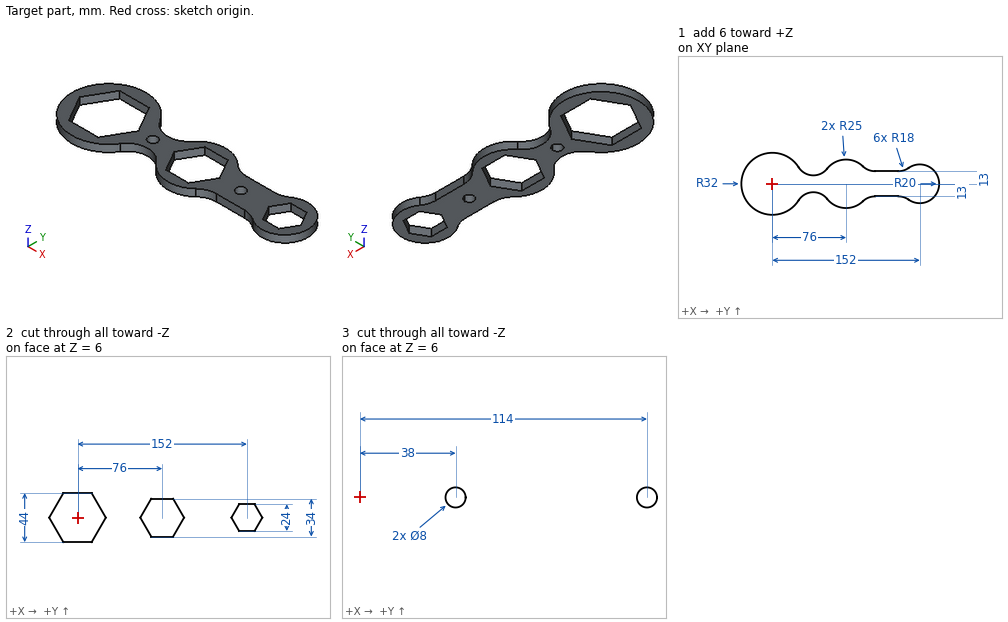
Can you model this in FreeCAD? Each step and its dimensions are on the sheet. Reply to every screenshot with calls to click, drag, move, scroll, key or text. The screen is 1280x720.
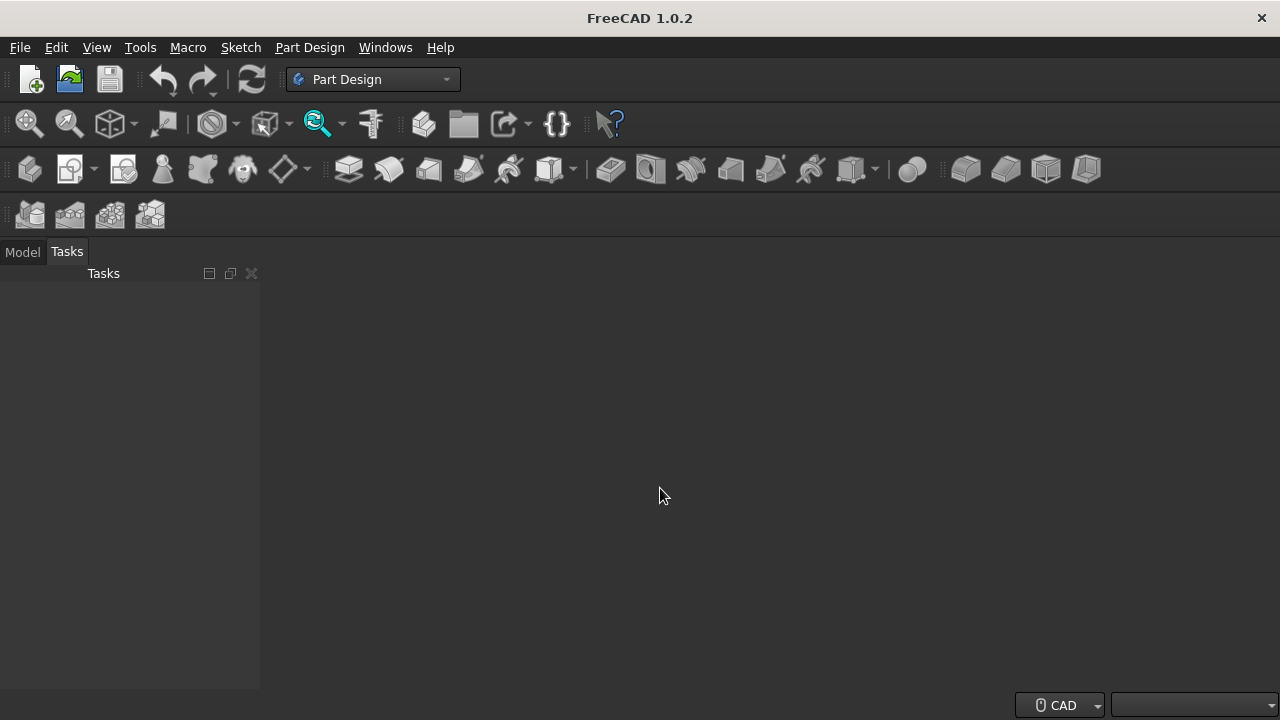
click(30, 80)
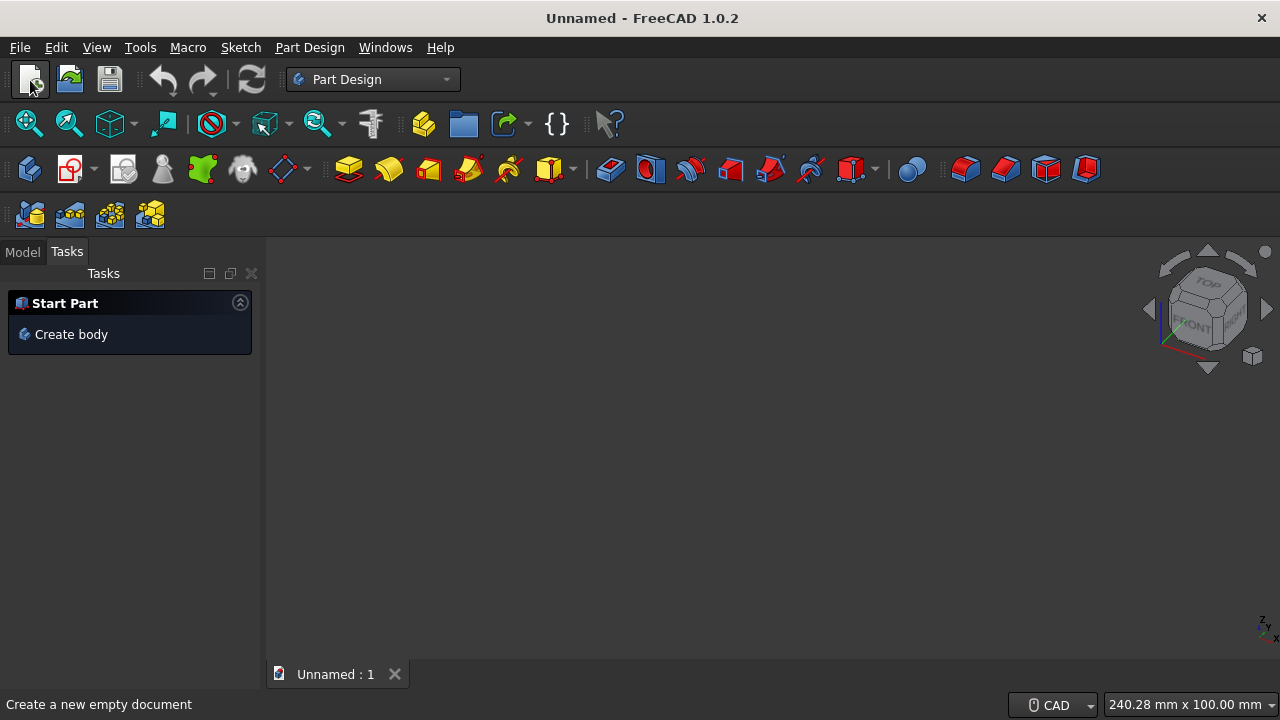
click(70, 170)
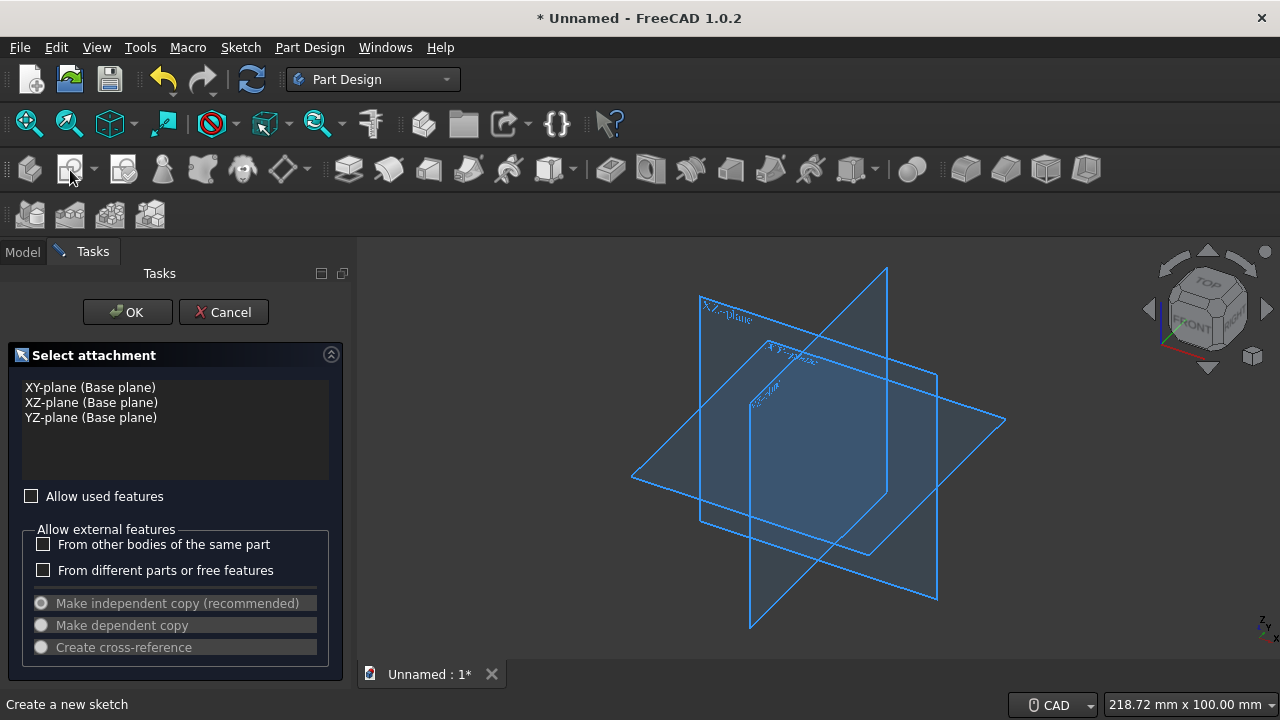
click(82, 388)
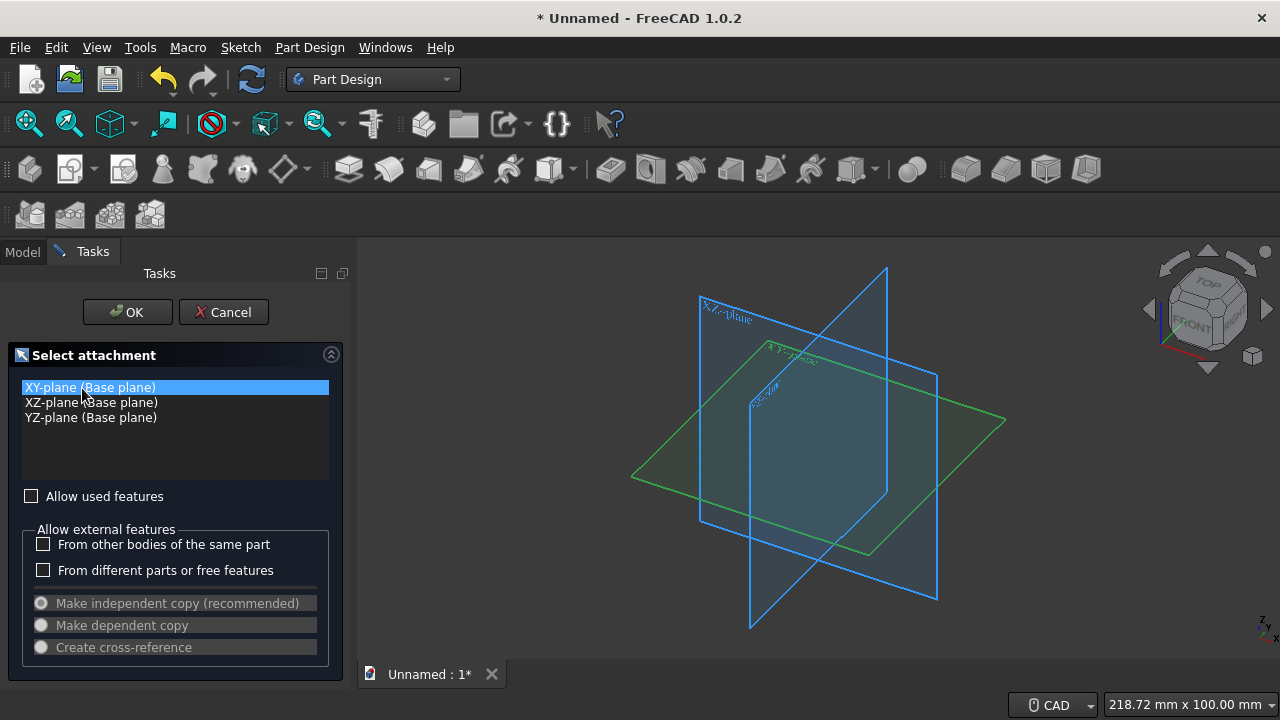
click(128, 312)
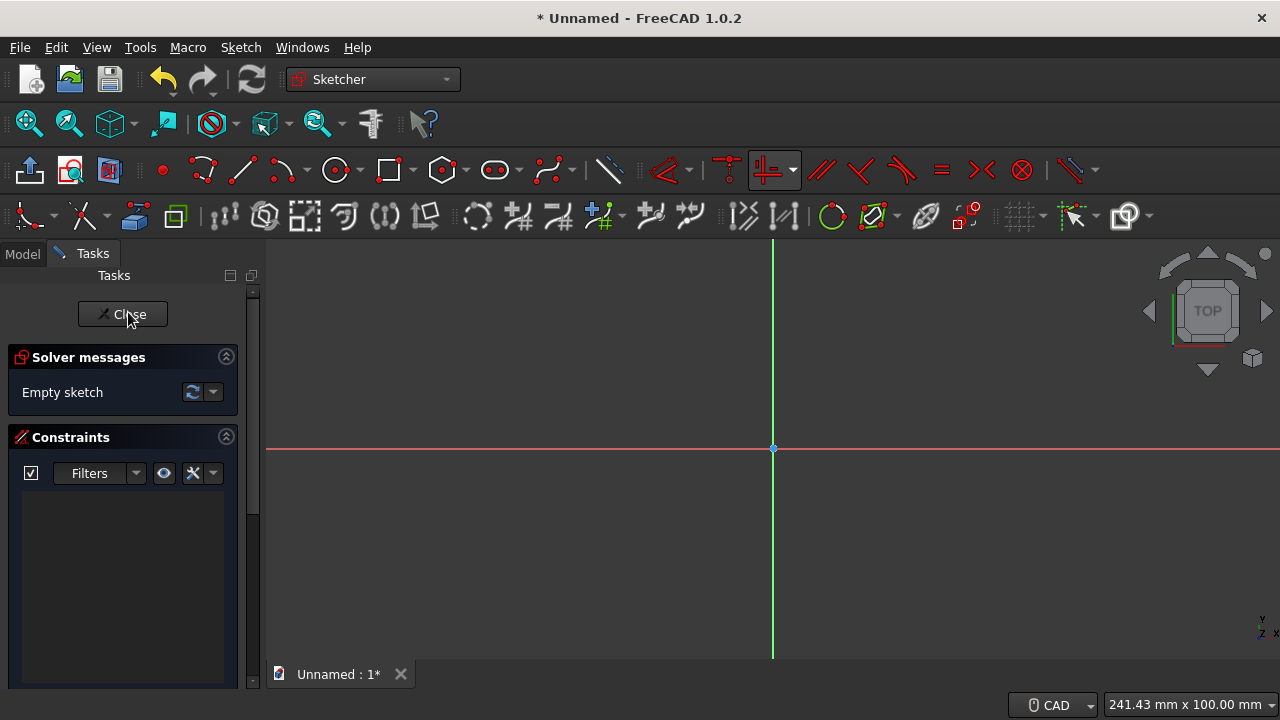
scroll(294, 449, down, 3)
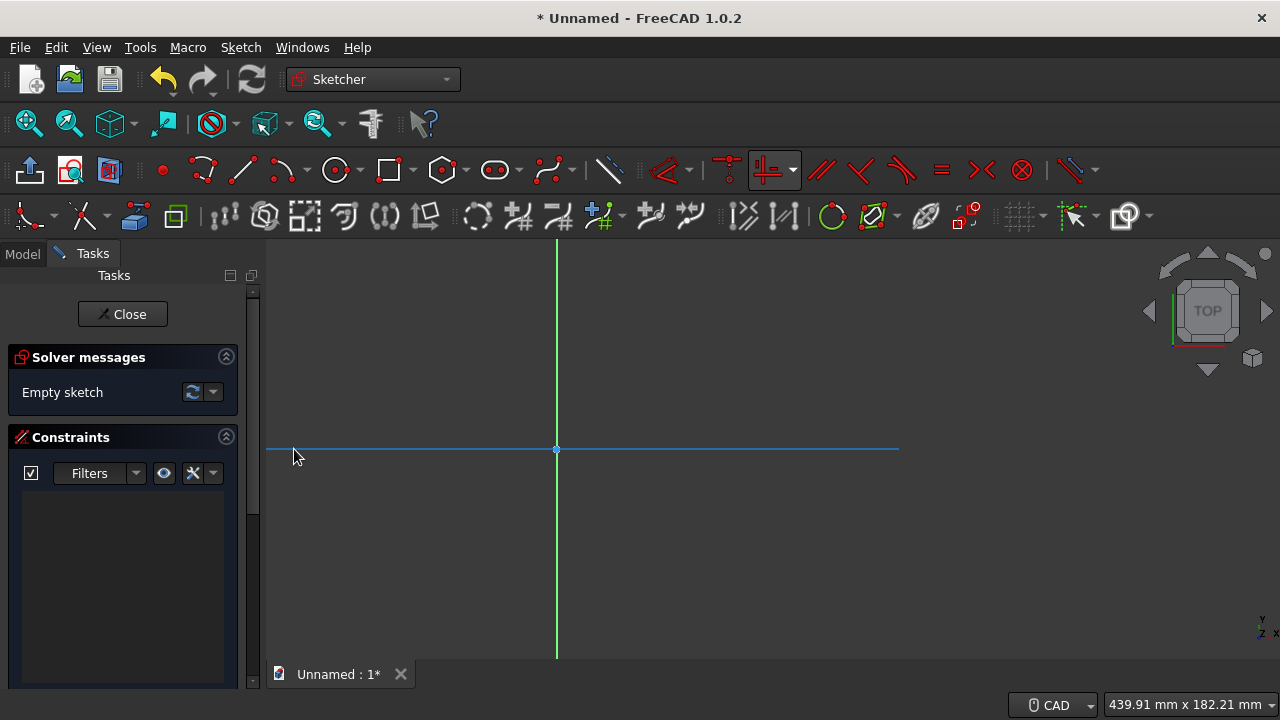
click(244, 170)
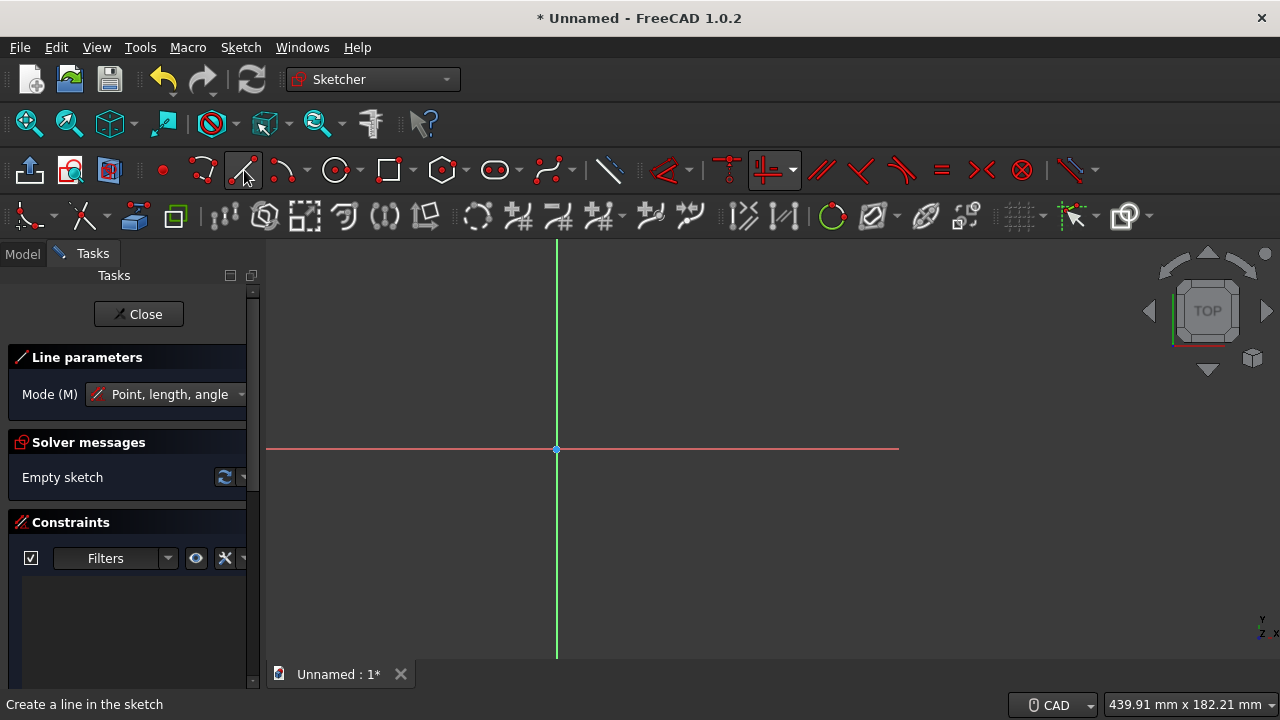
click(801, 479)
click(857, 479)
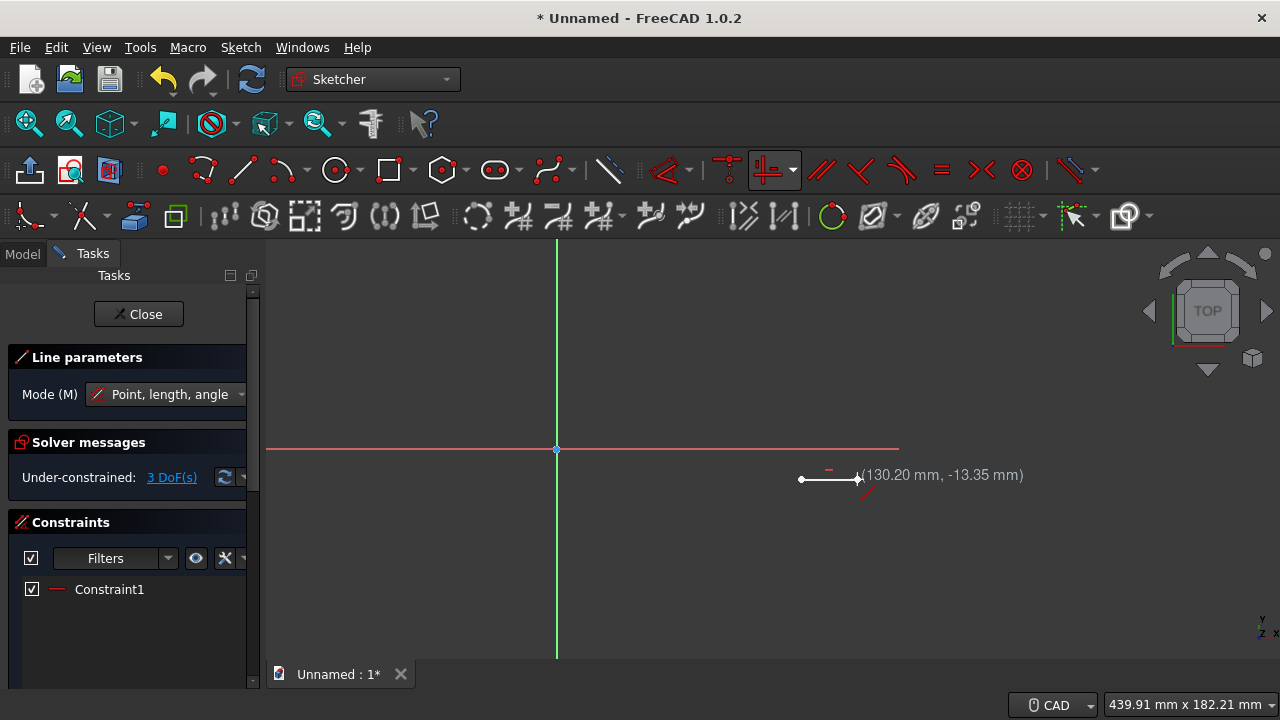
click(857, 419)
click(801, 419)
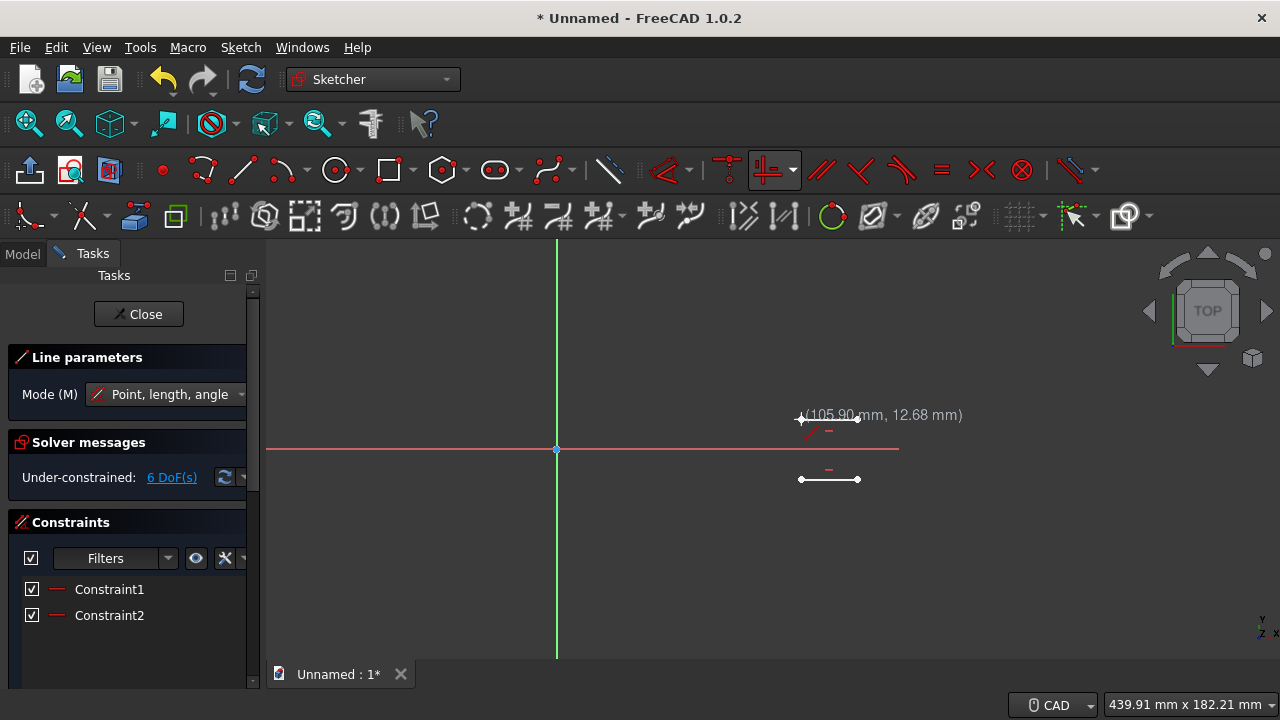
click(310, 170)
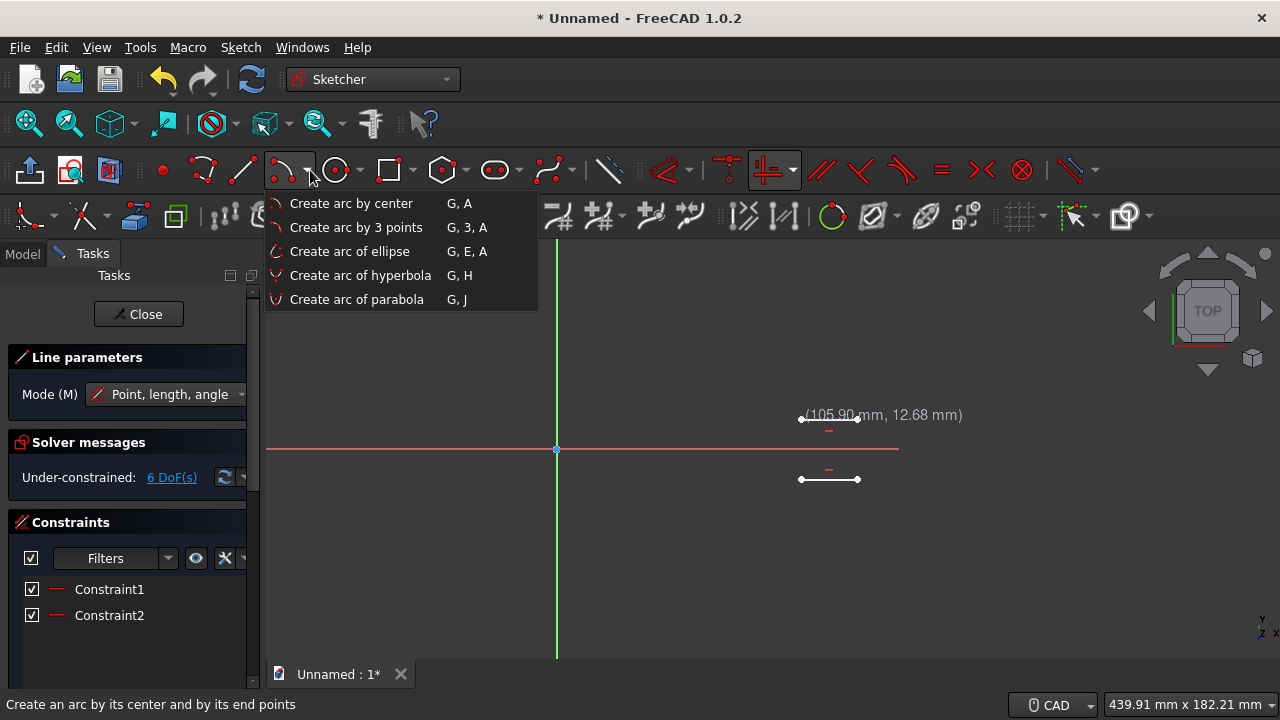
click(402, 227)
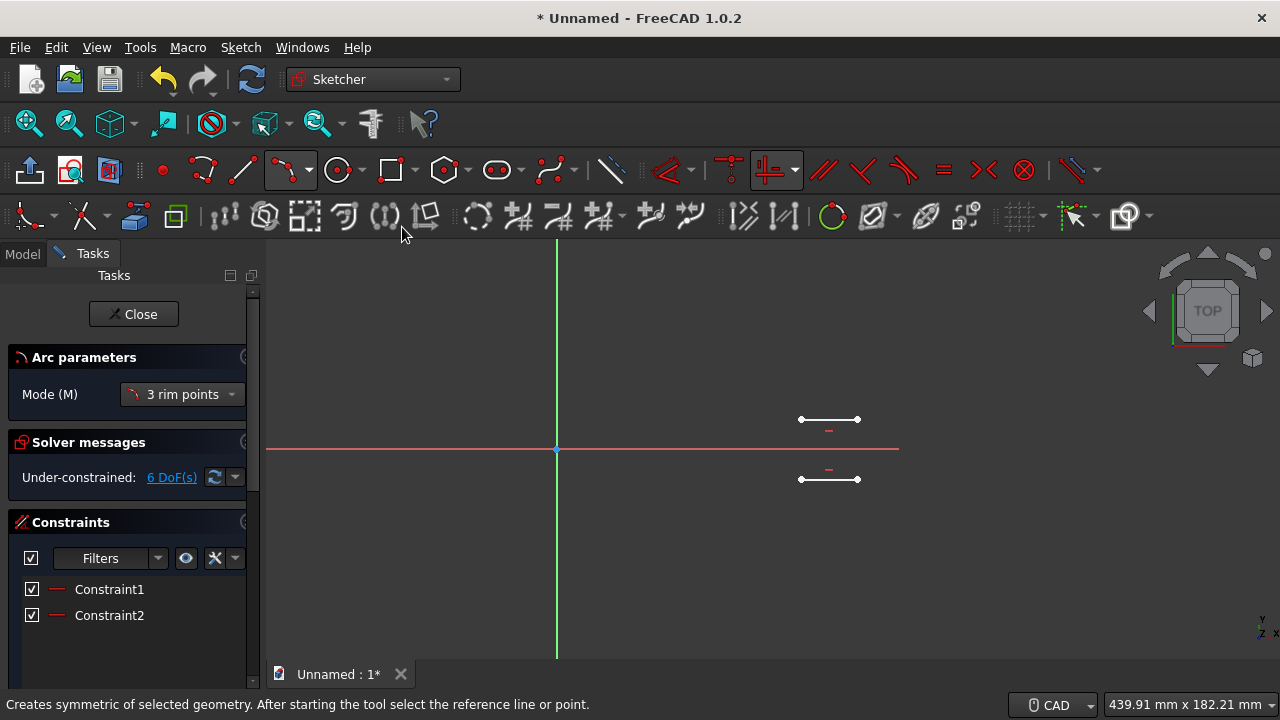
click(857, 480)
click(881, 487)